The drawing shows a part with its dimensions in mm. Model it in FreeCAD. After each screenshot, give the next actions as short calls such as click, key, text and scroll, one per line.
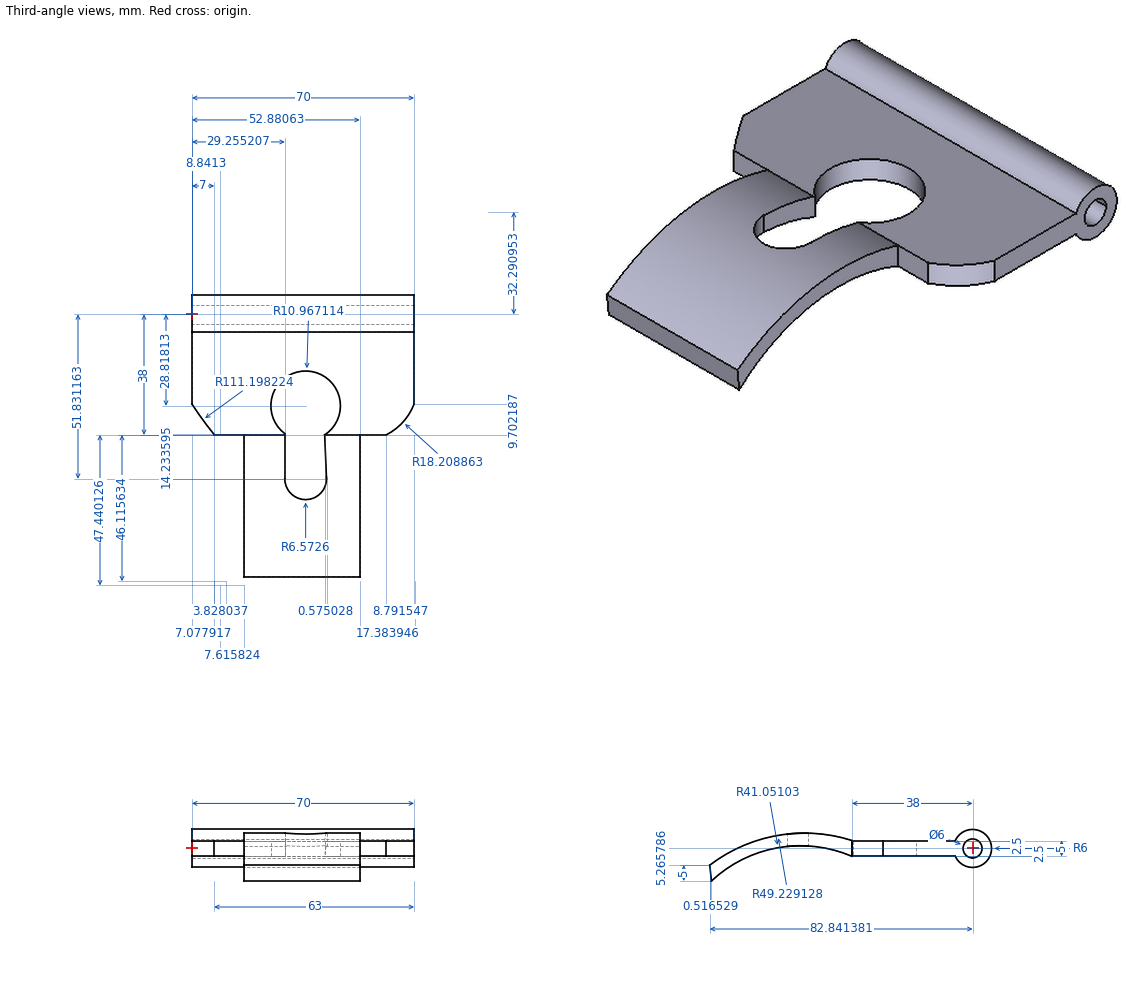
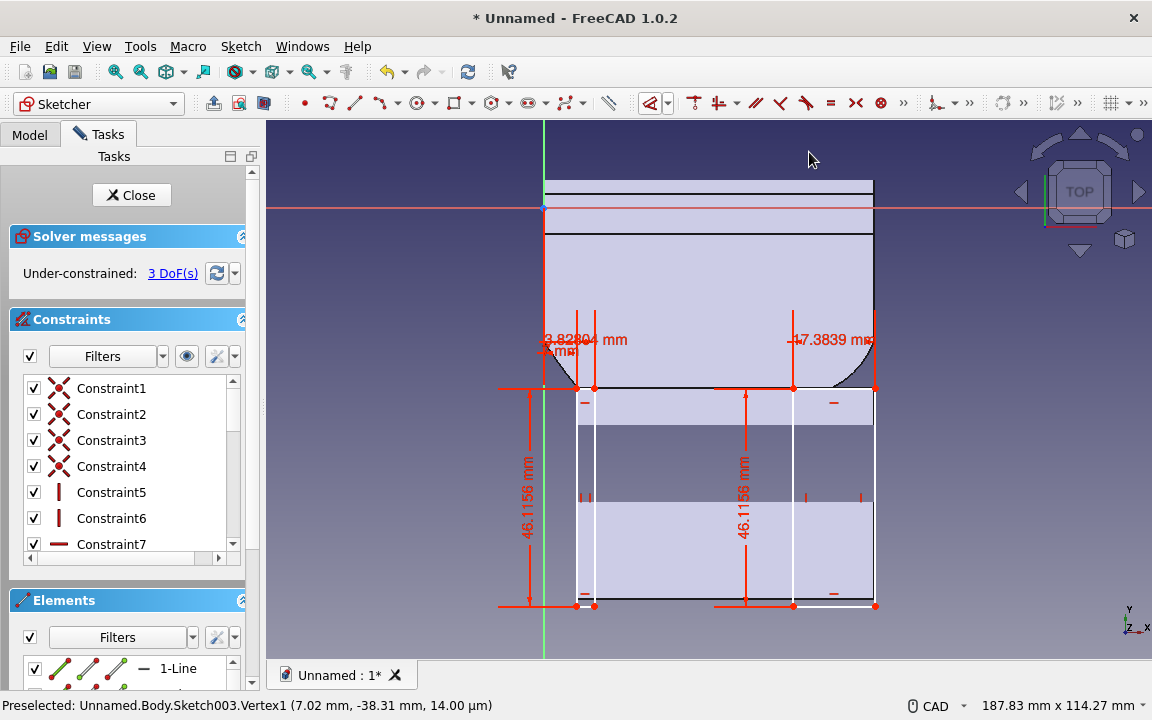
click(577, 389)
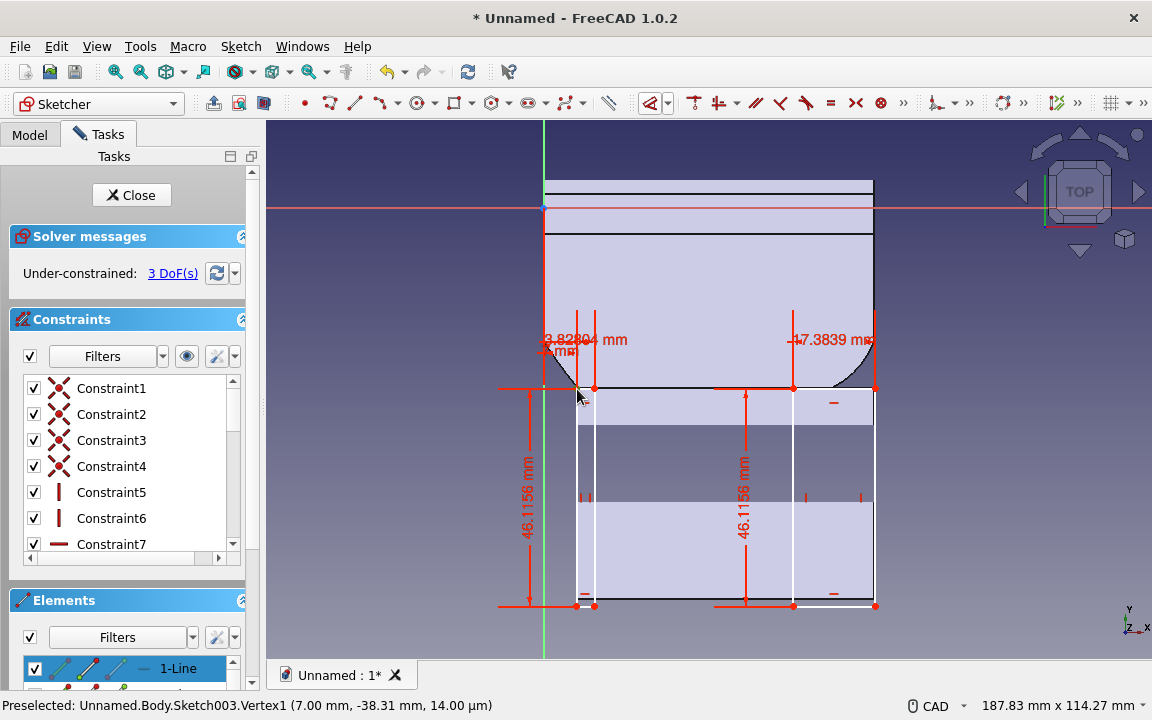
click(668, 104)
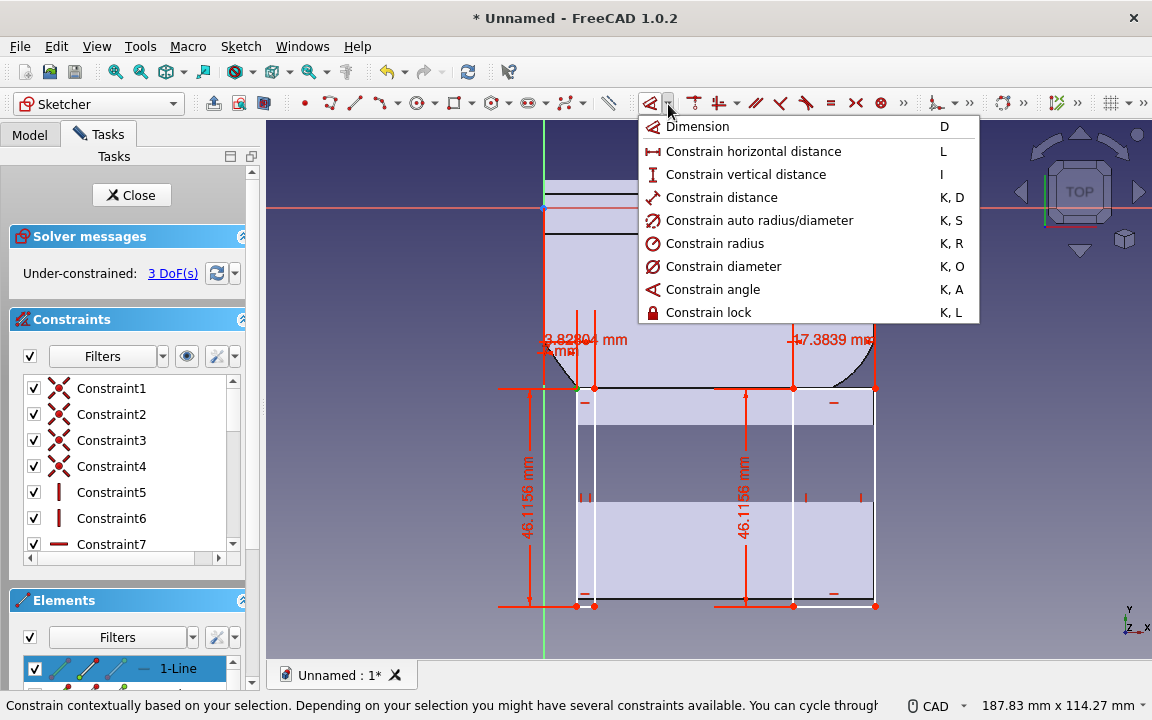
click(809, 174)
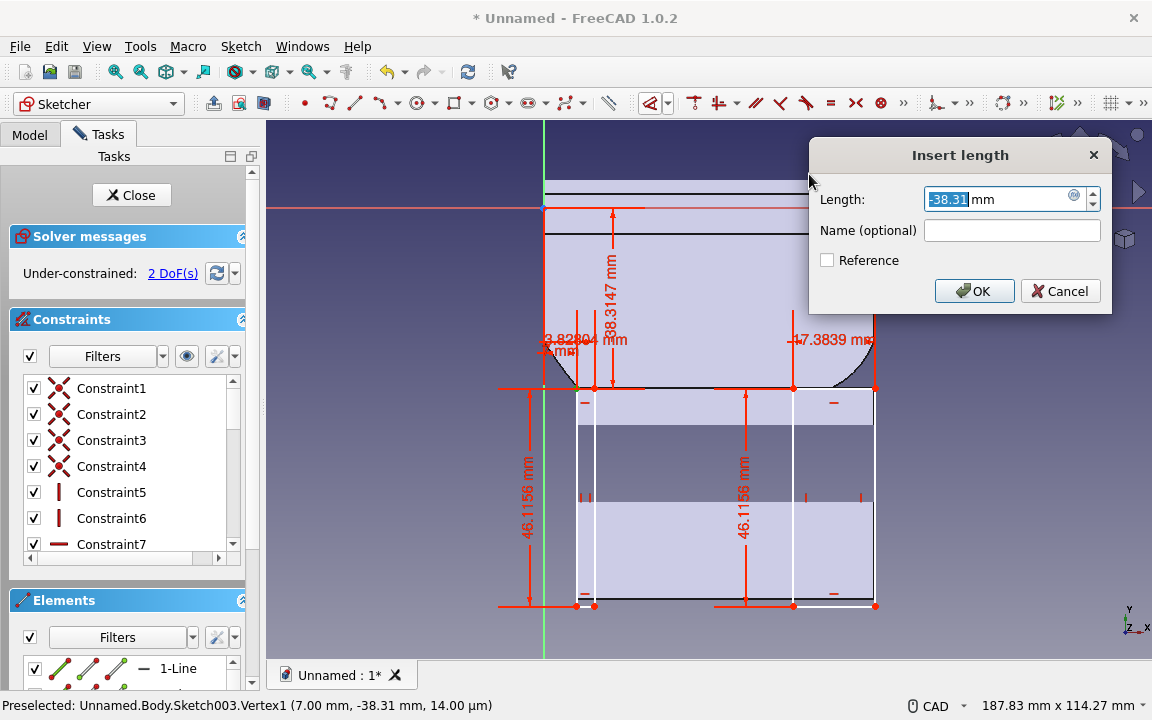
text(-38)
key(Return)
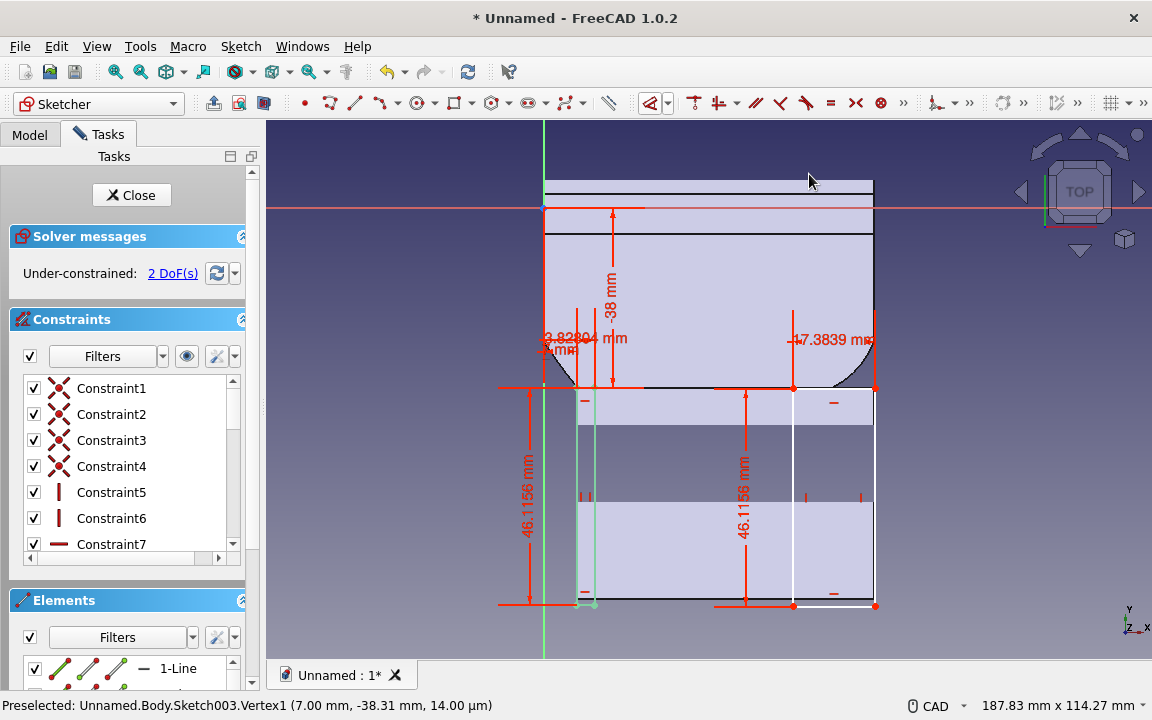
click(793, 389)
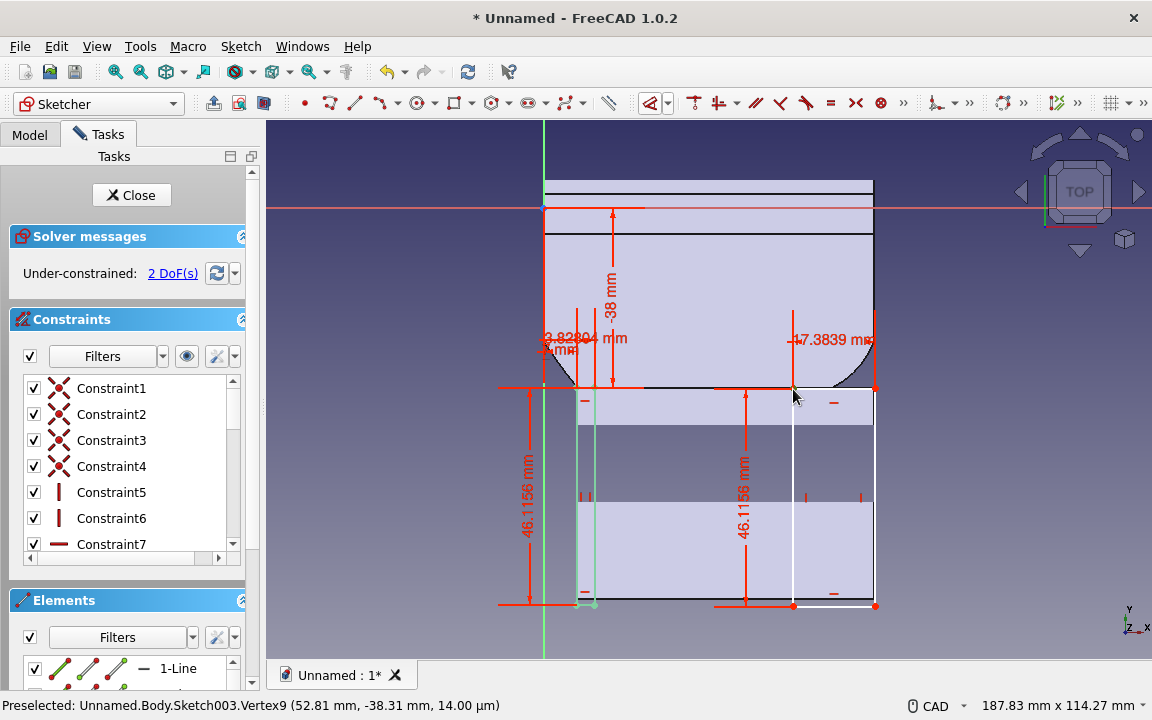
click(668, 104)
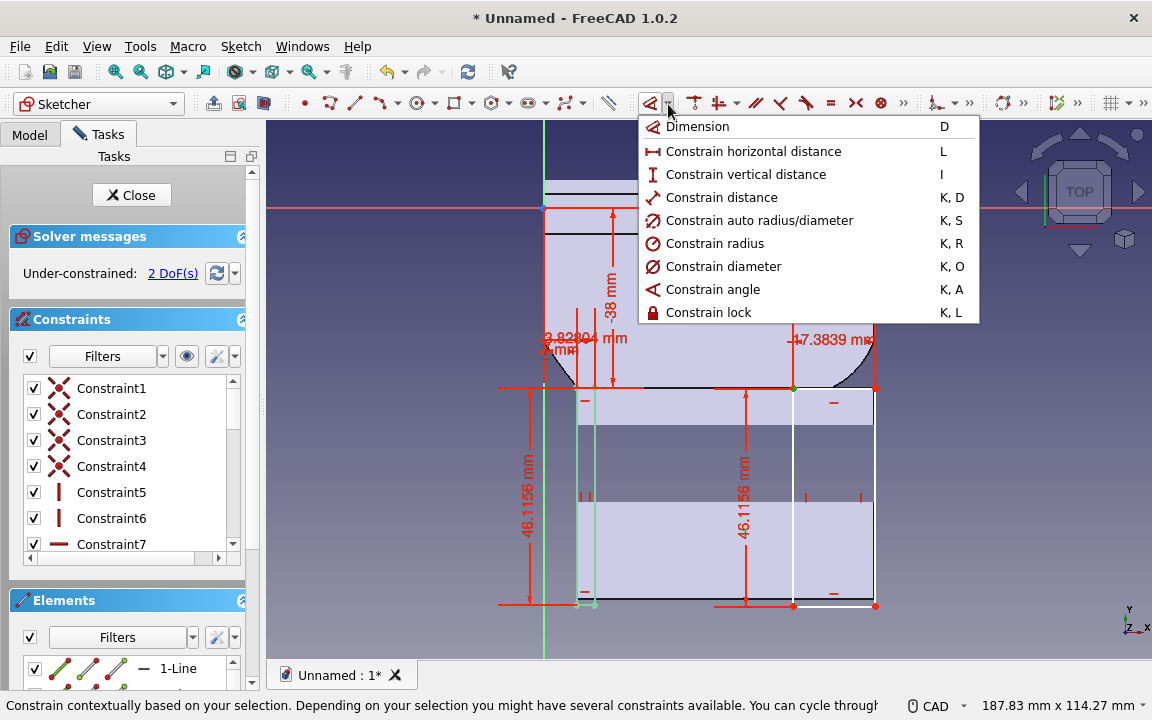
click(809, 174)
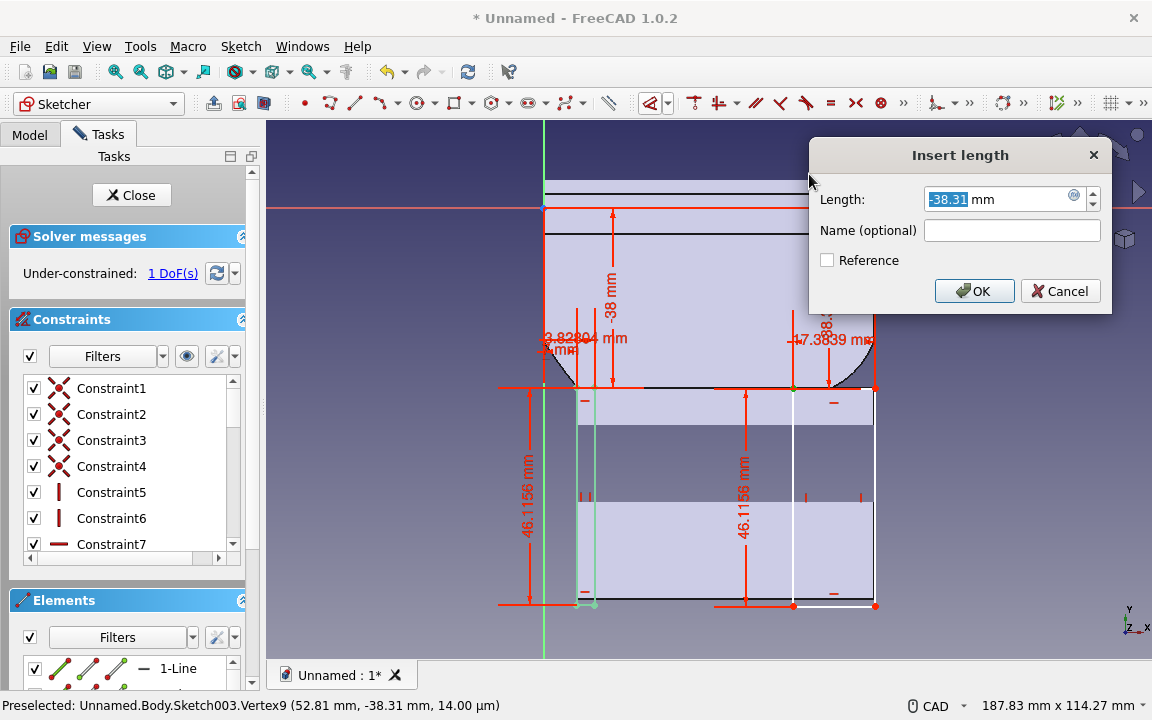
text(-38)
key(Return)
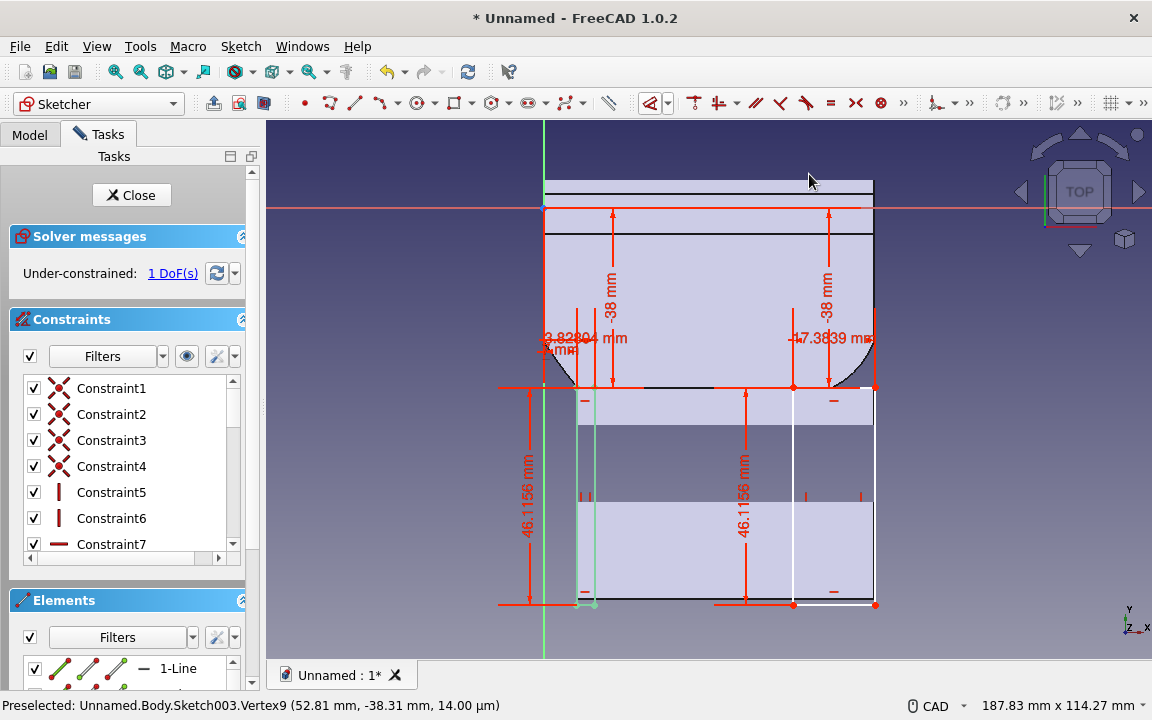
click(793, 388)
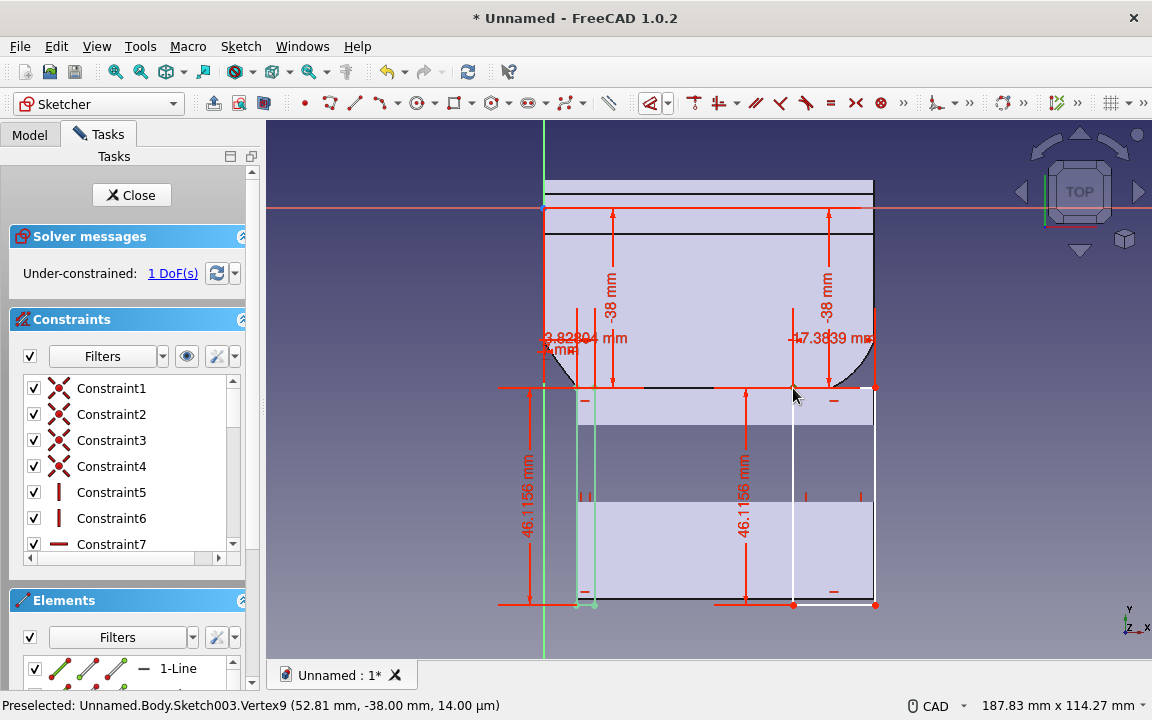
click(668, 104)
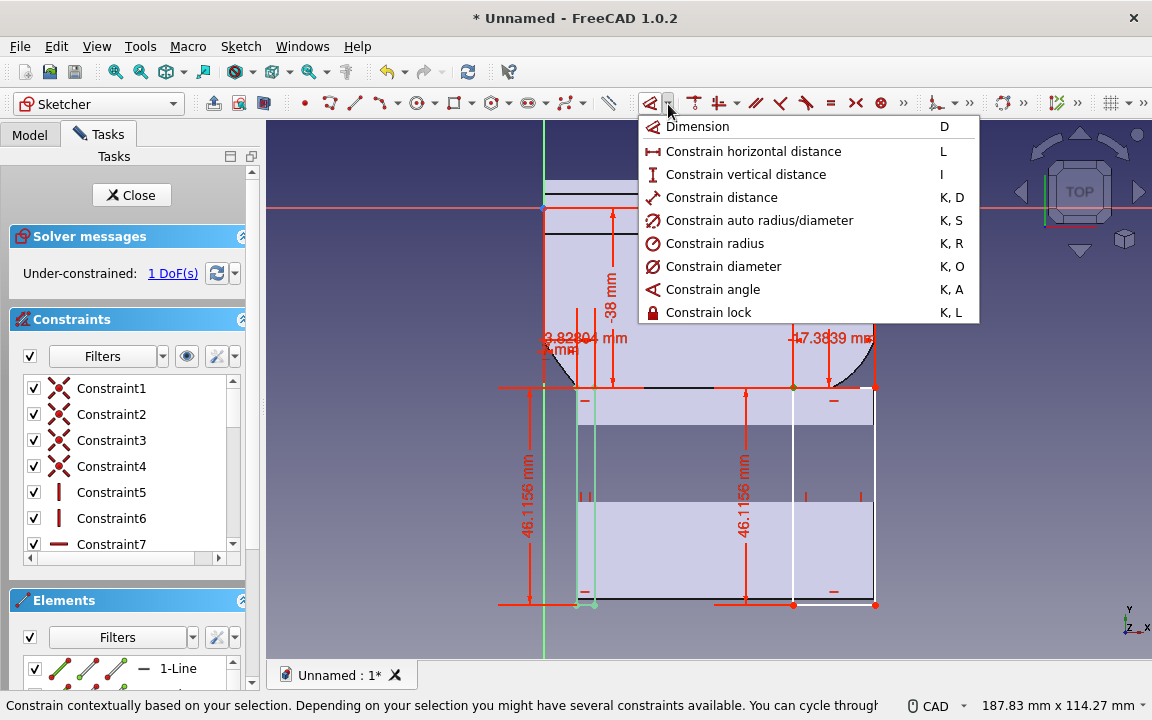
click(809, 152)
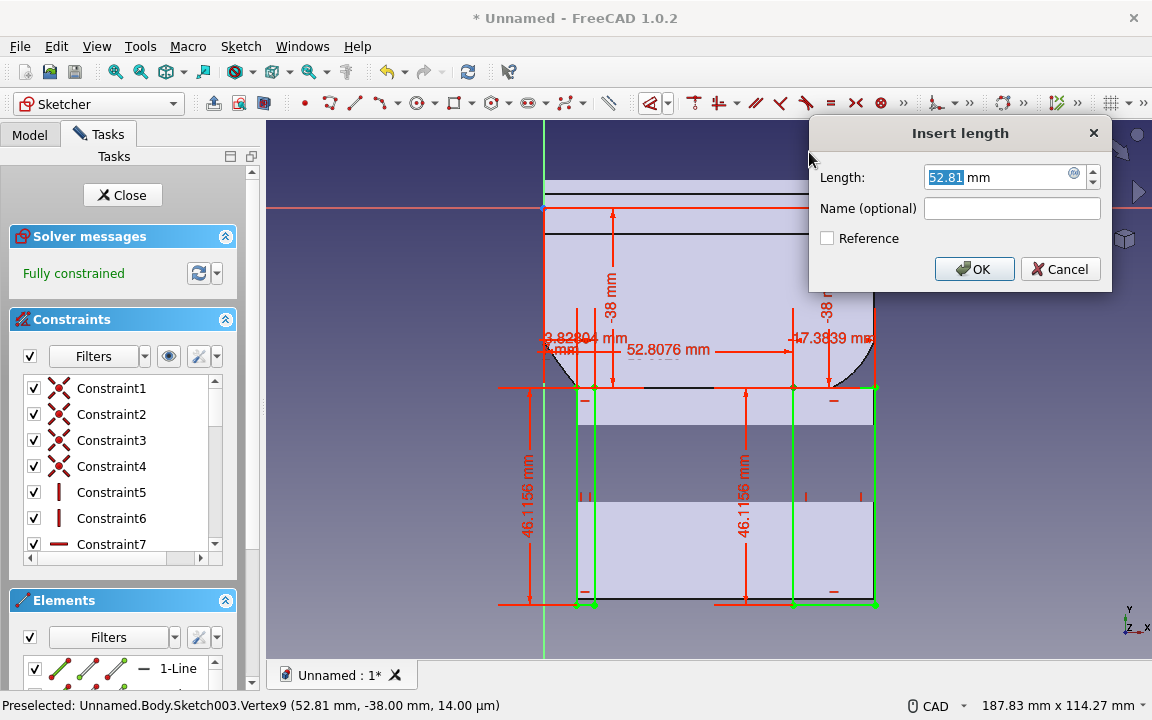
text(52.88063)
key(Return)